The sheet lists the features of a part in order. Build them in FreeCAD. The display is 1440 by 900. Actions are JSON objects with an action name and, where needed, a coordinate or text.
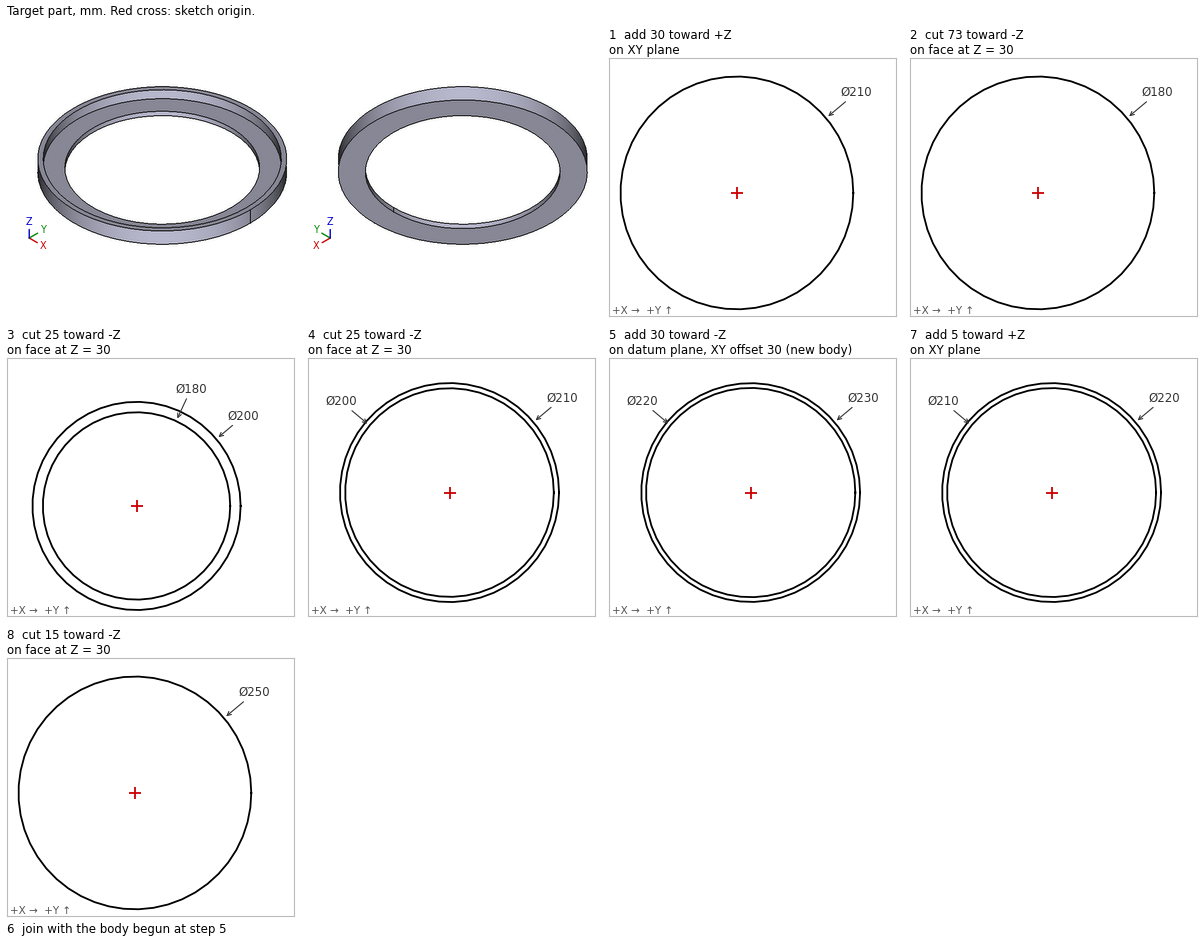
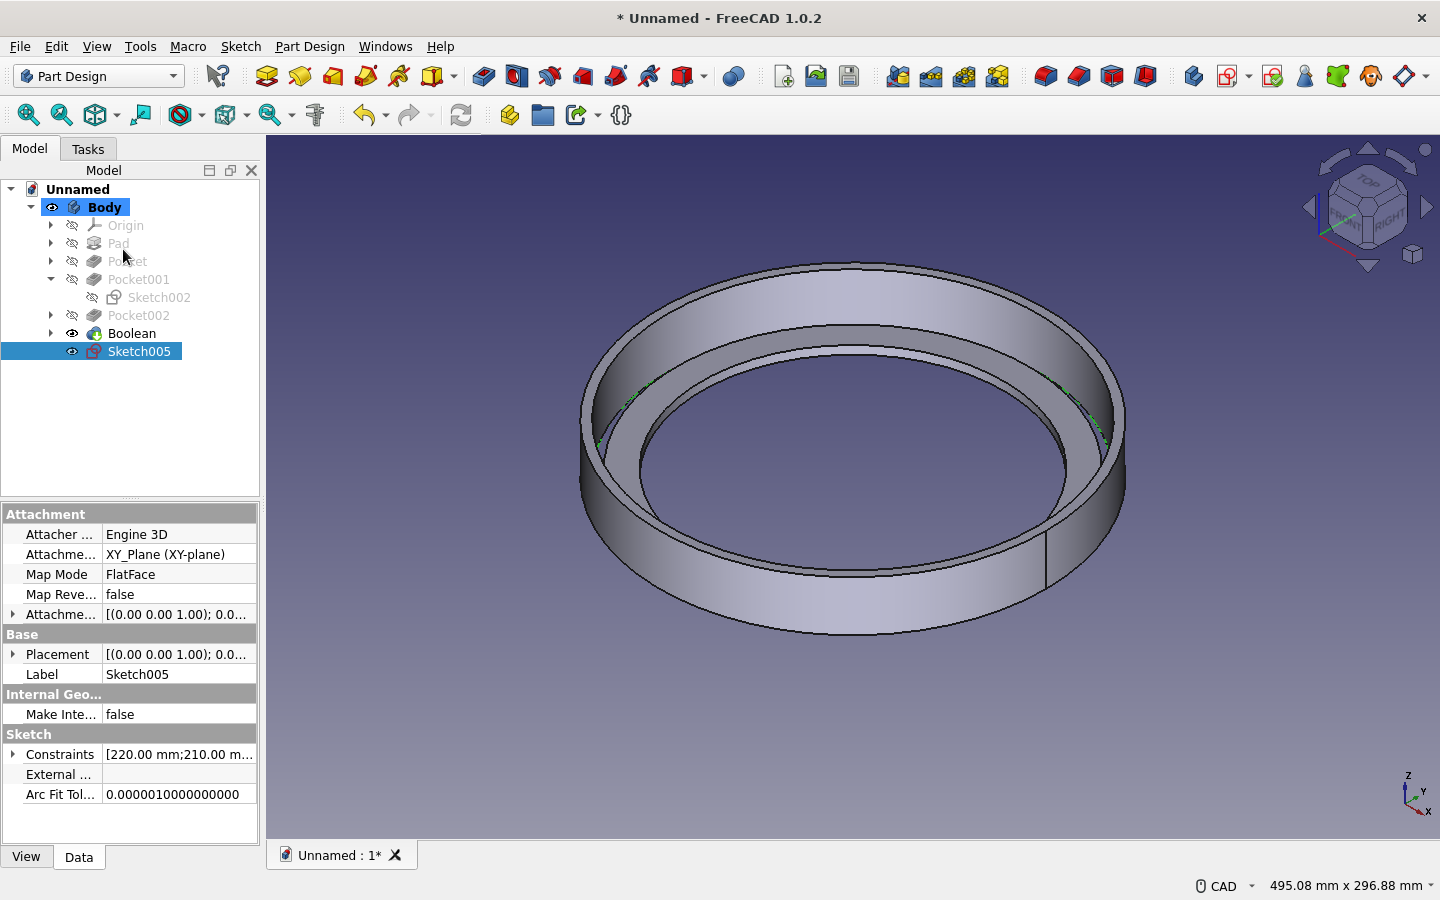
{"action": "left_click", "coordinate": [267, 76]}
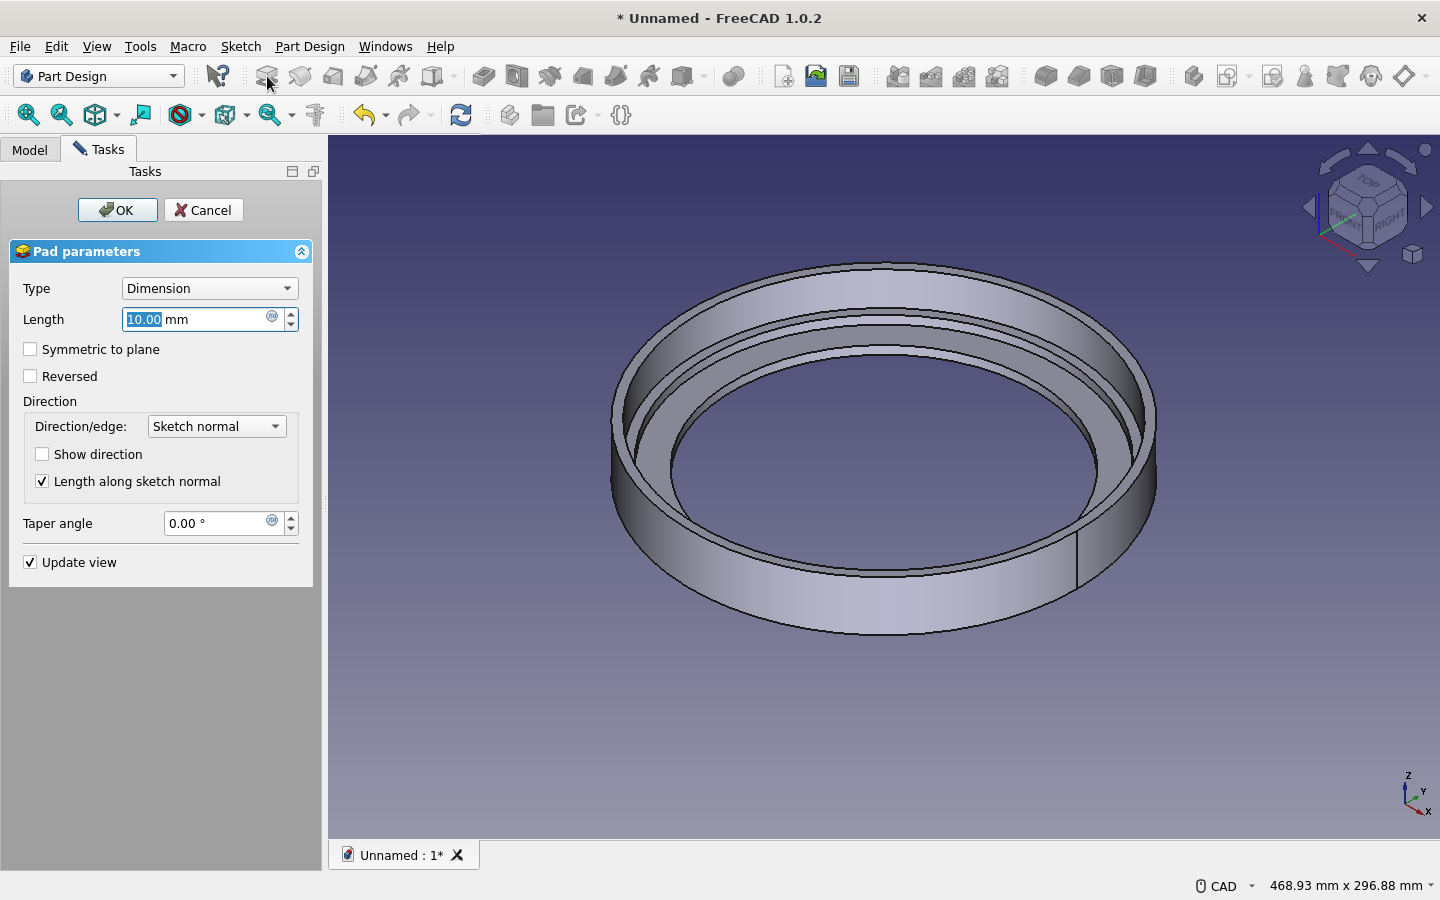
{"action": "type", "text": "5"}
{"action": "key", "text": "Tab"}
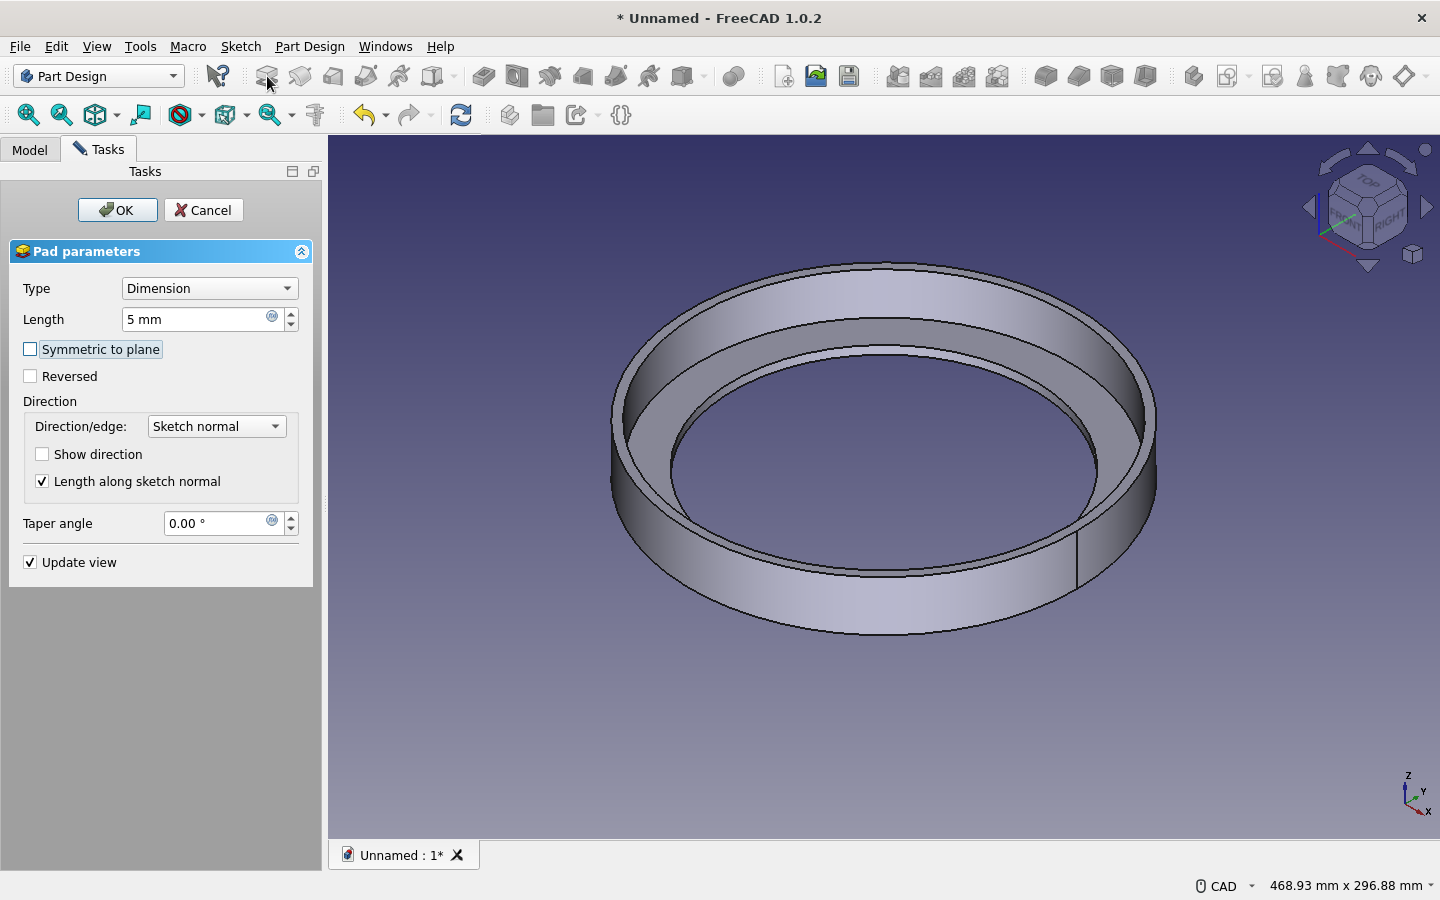
{"action": "left_click", "coordinate": [118, 210]}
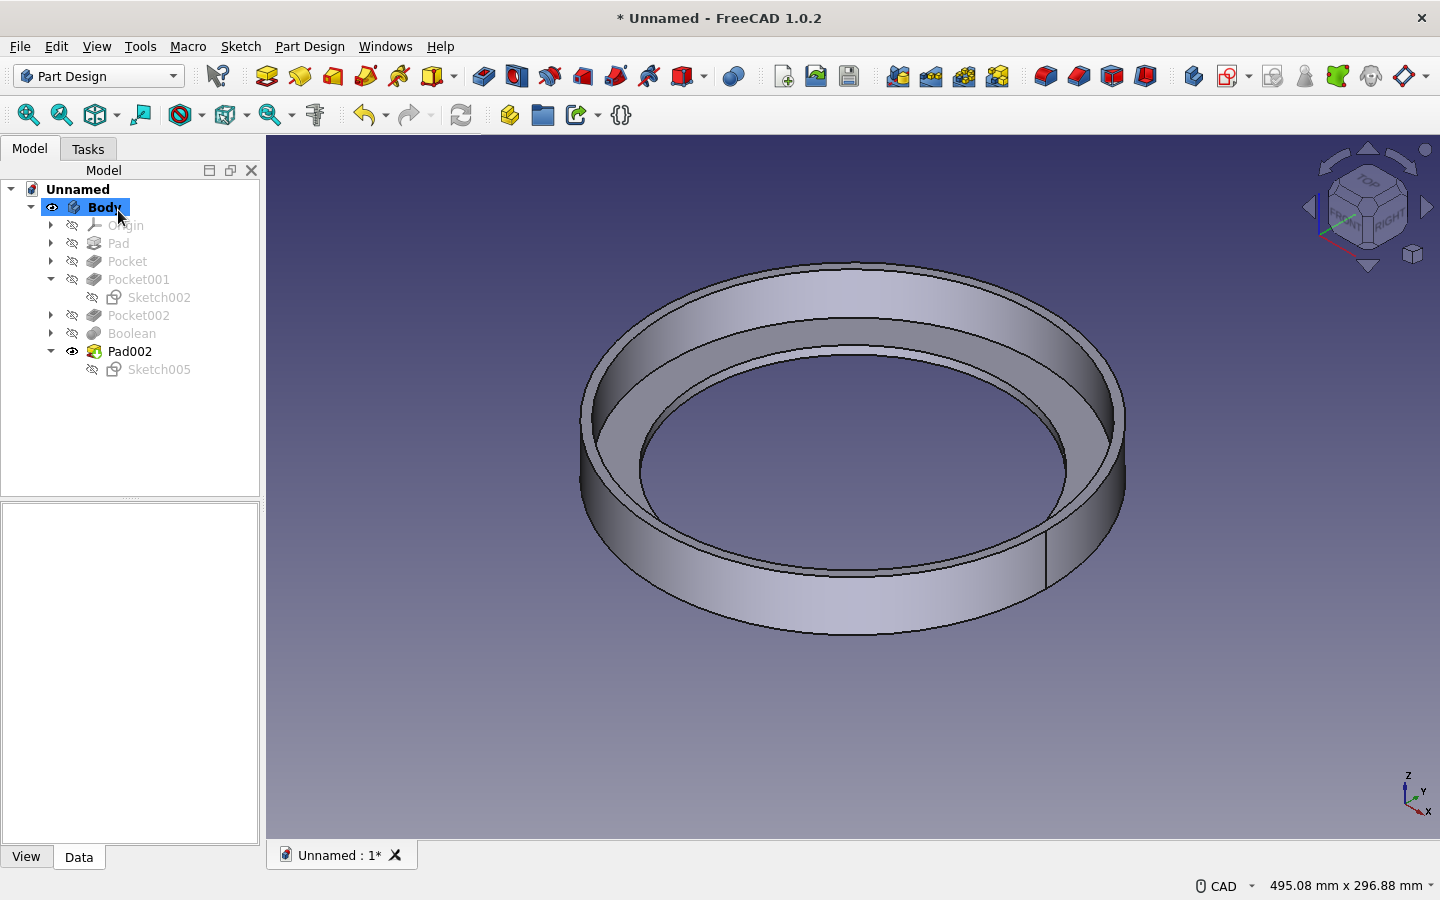
{"action": "scroll", "coordinate": [741, 560], "scroll_direction": "up", "scroll_amount": 6}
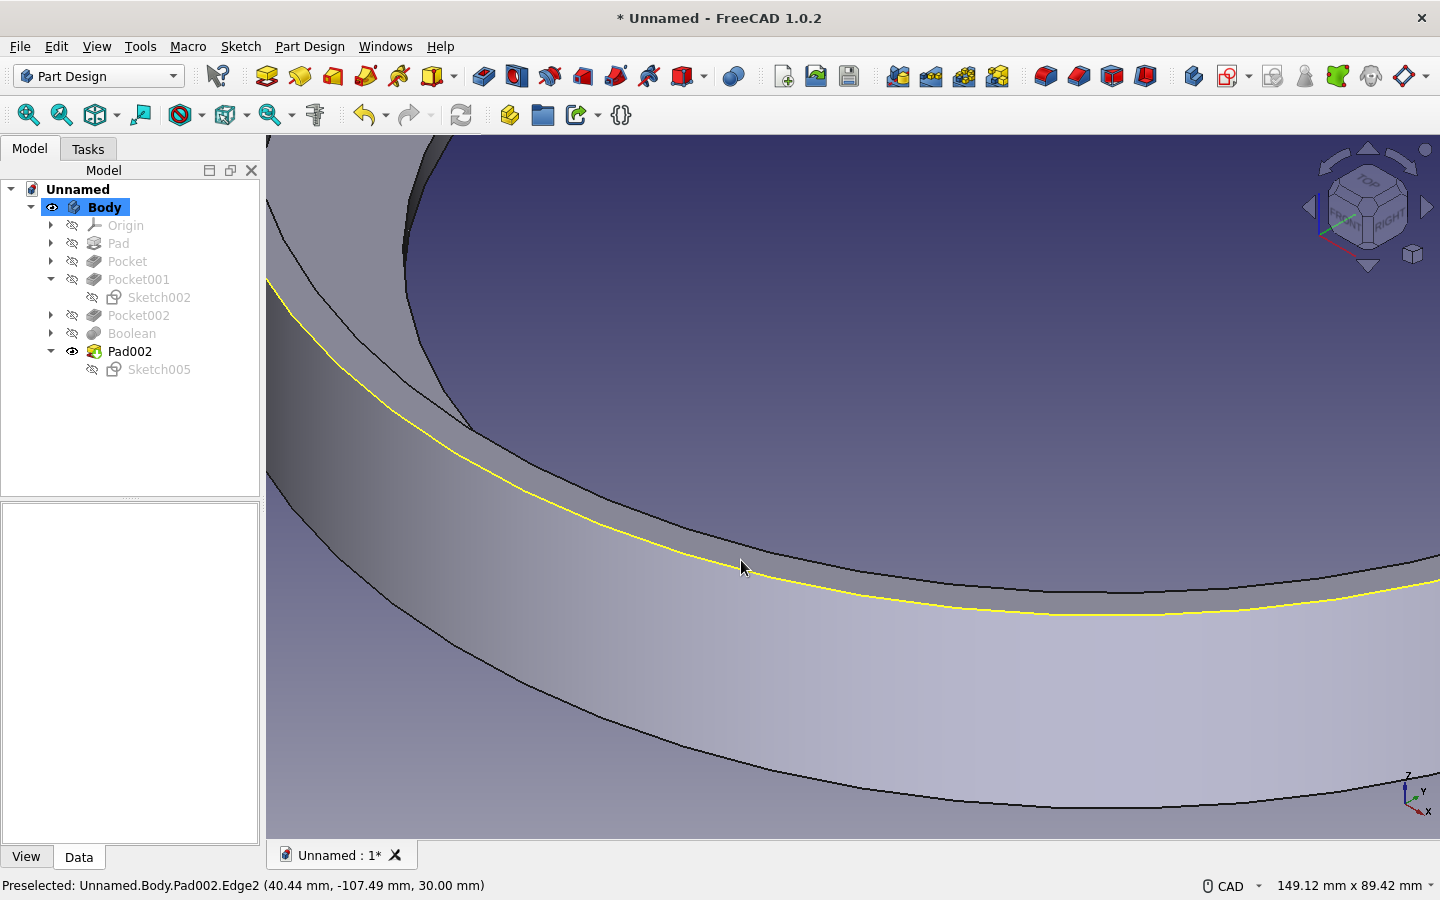
{"action": "left_click", "coordinate": [29, 116]}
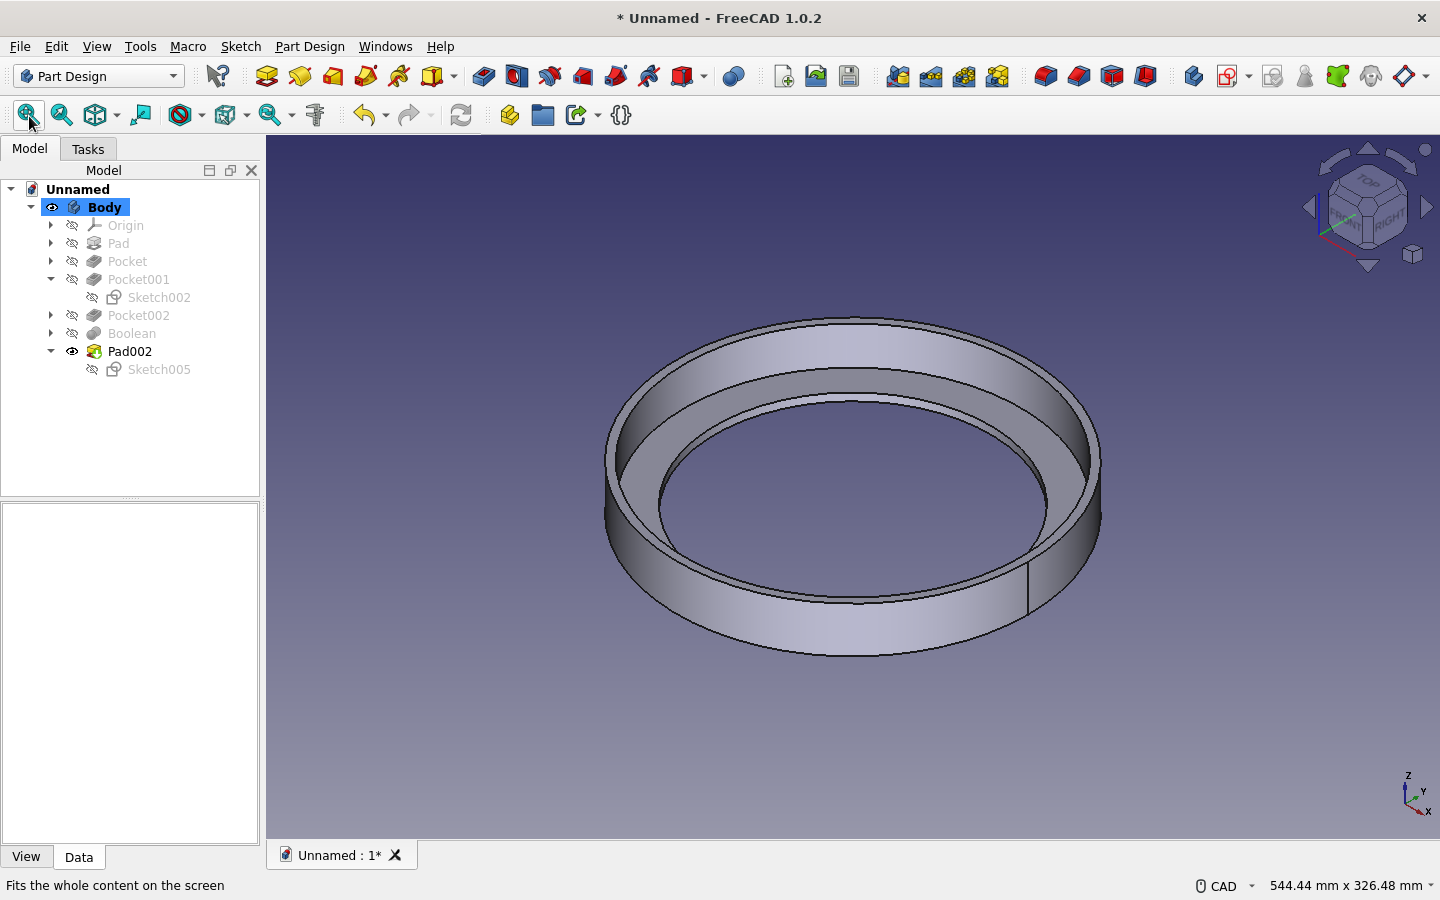
{"action": "key", "text": "2"}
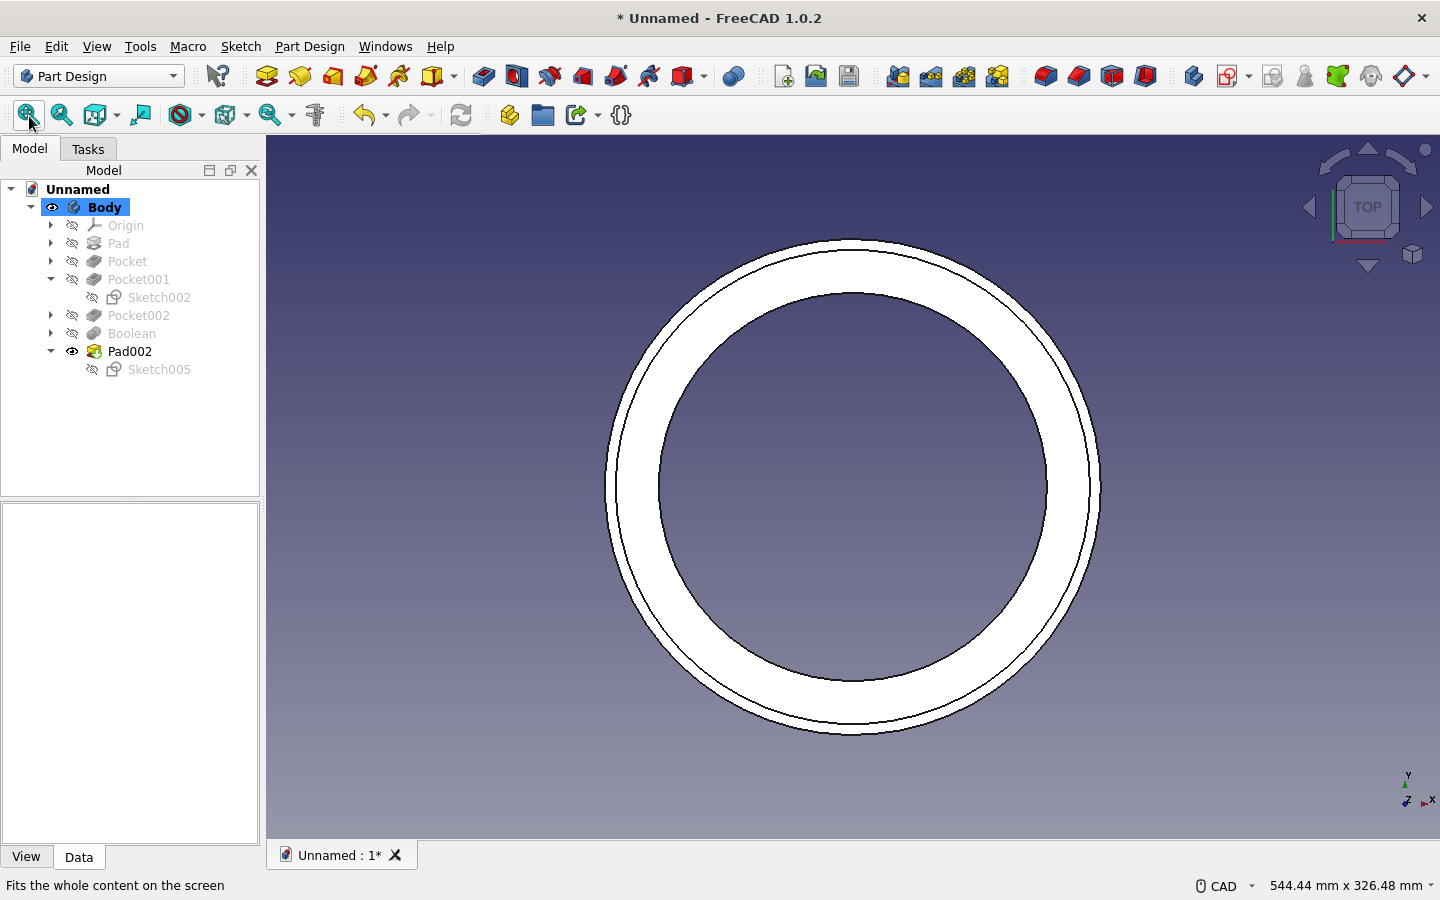
{"action": "scroll", "coordinate": [938, 715], "scroll_direction": "up", "scroll_amount": 6}